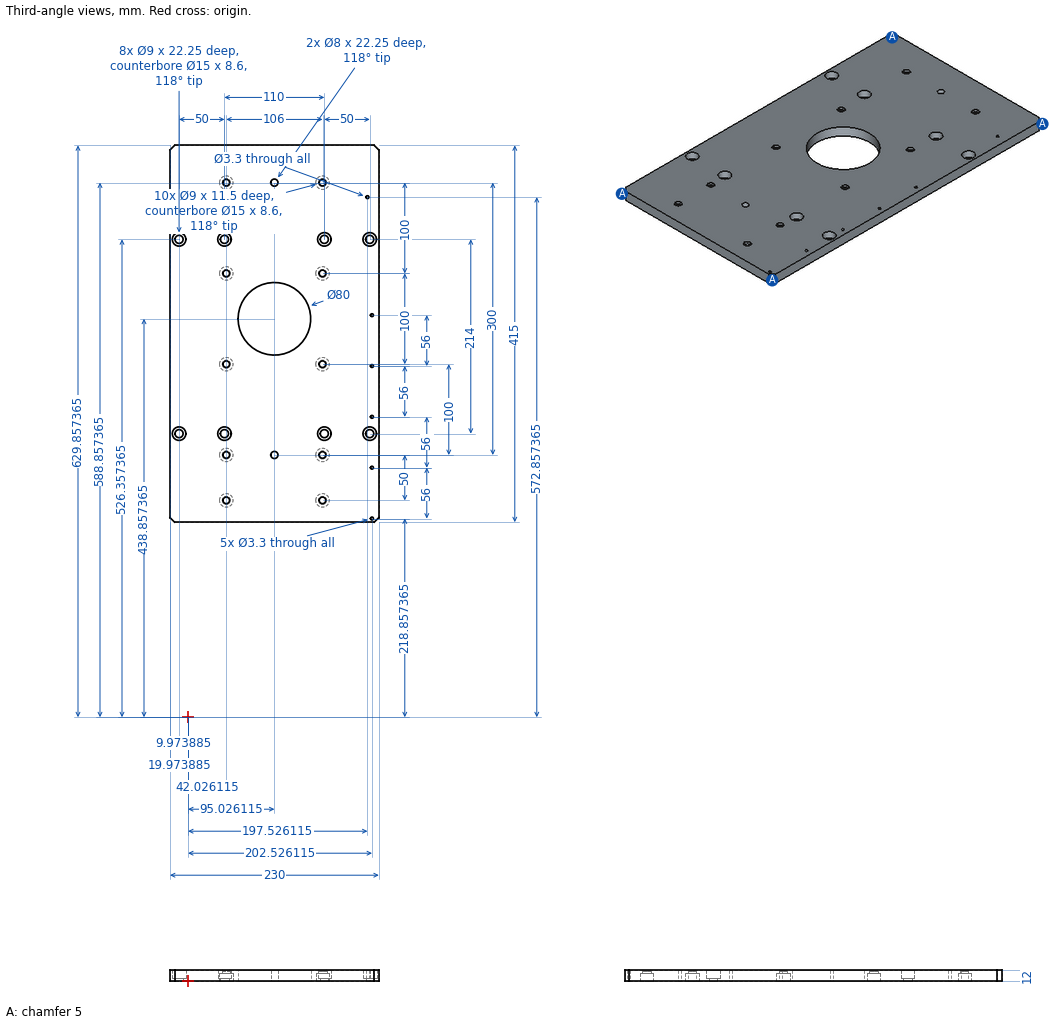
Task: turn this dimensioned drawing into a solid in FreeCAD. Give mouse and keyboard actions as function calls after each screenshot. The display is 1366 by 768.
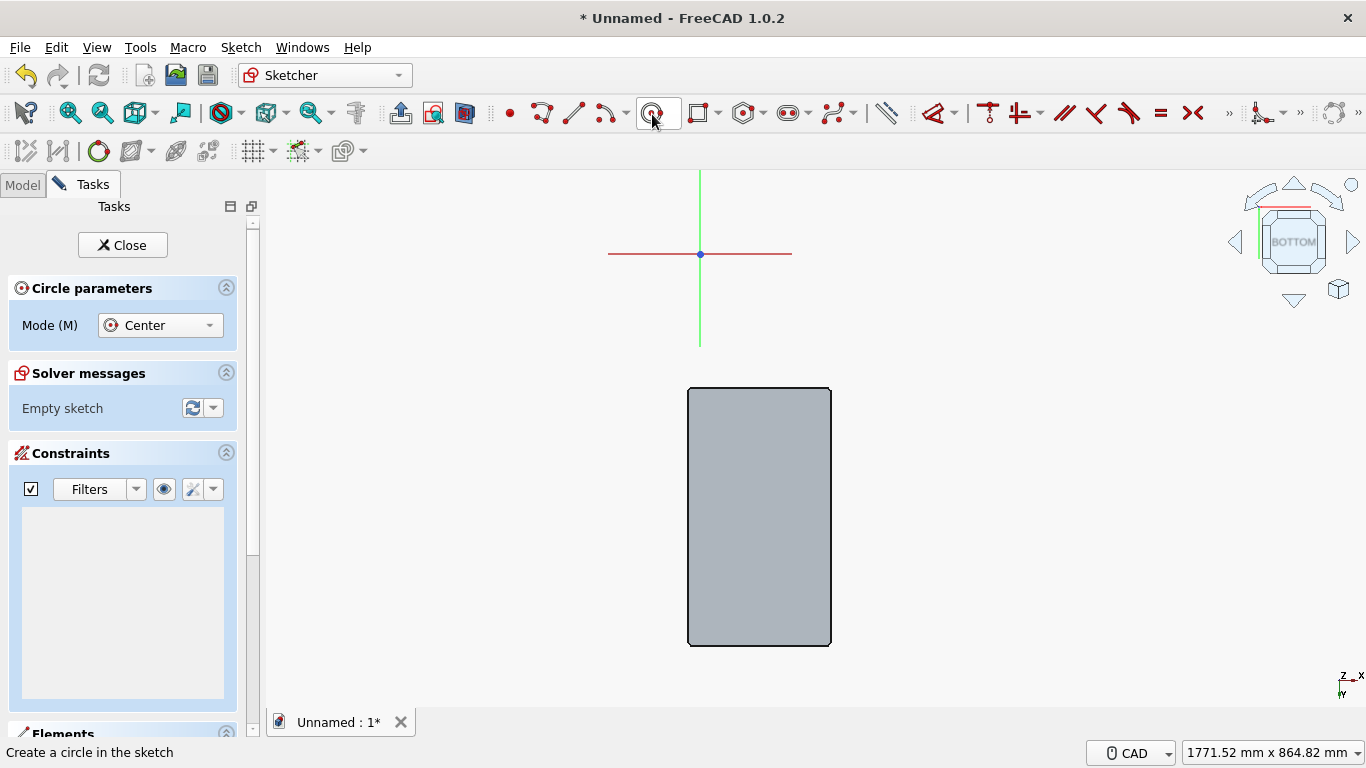
scroll(792, 620, up, 11)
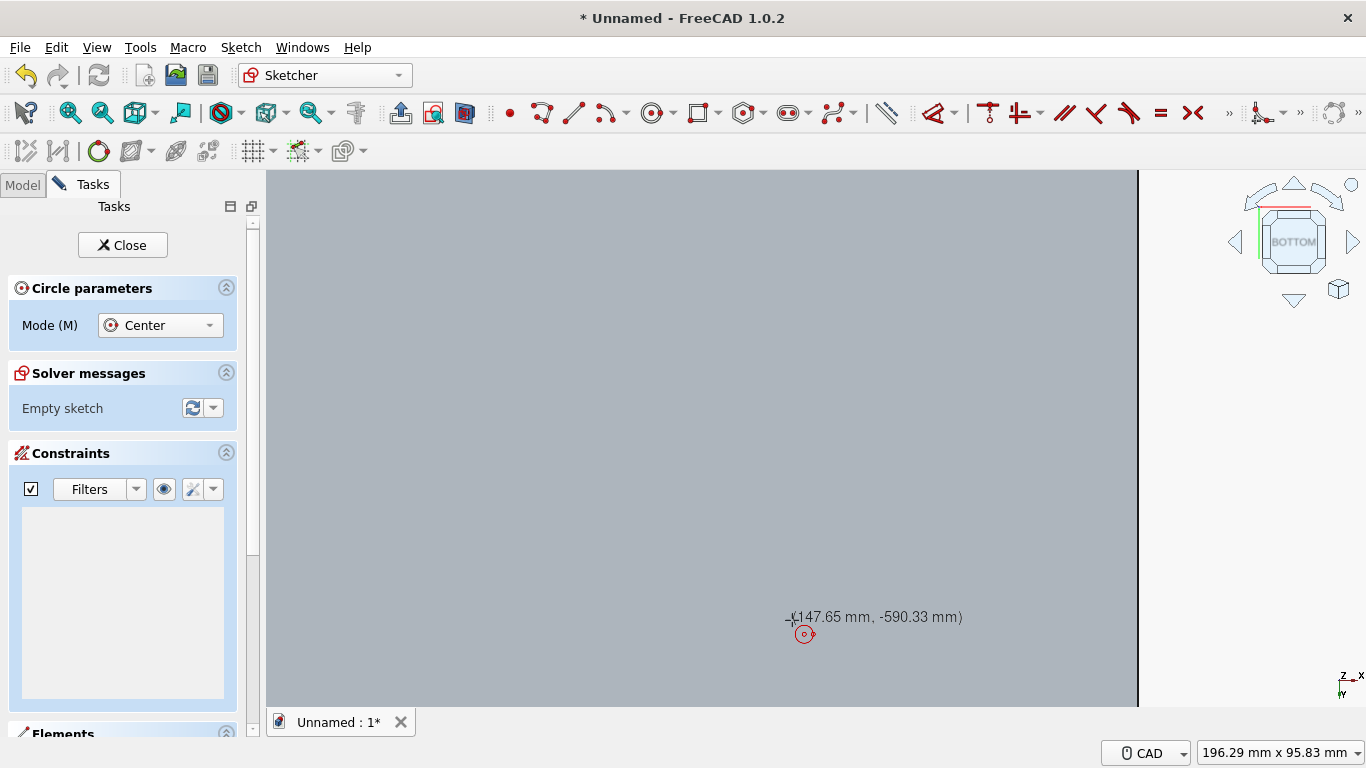
scroll(792, 621, down, 11)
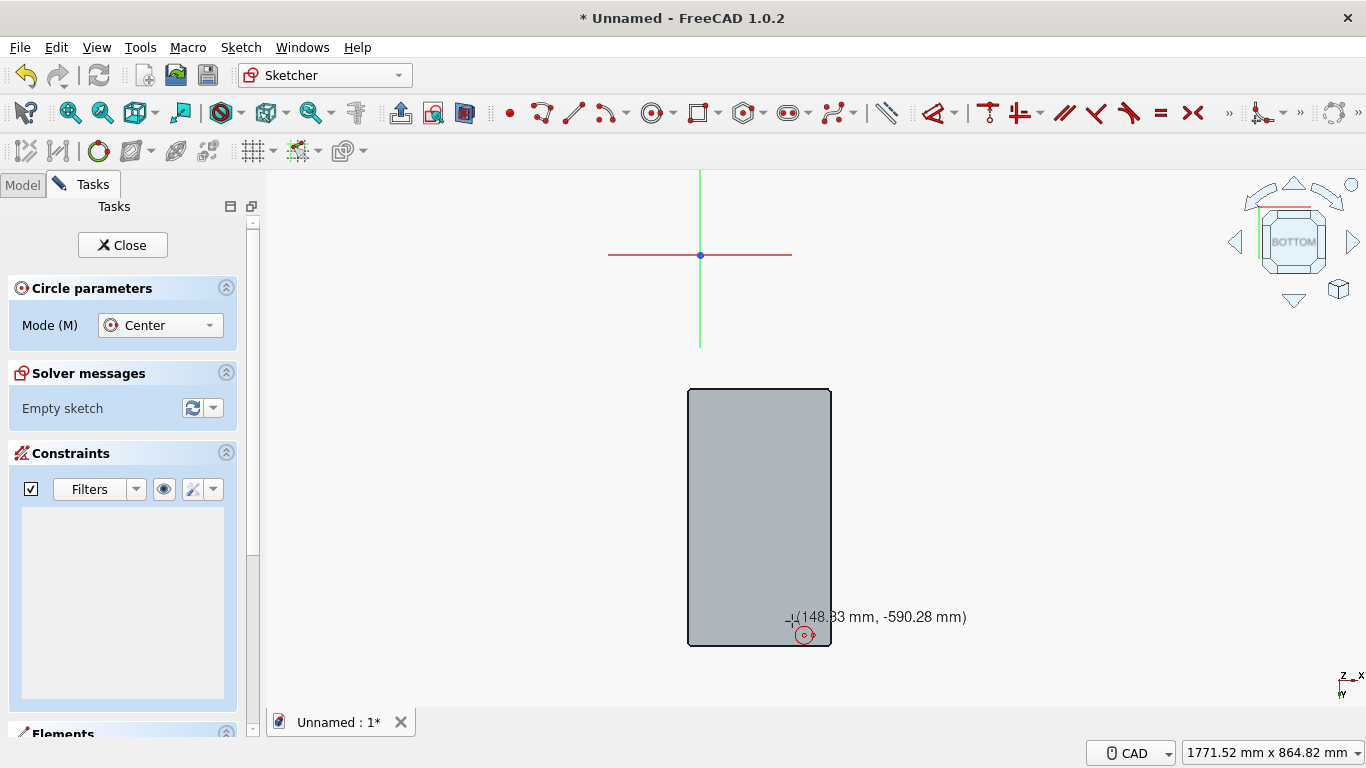
click(792, 621)
move(794, 619)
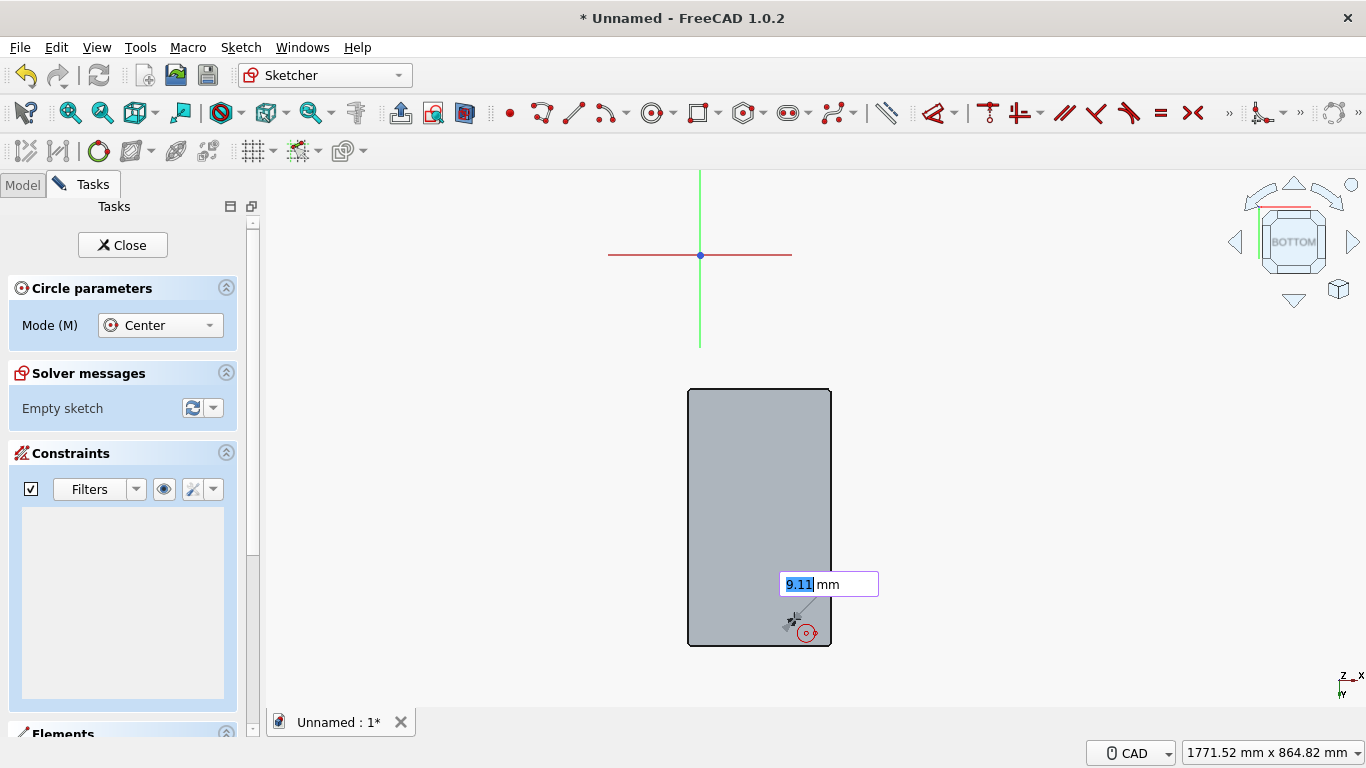
text(9)
key(Return)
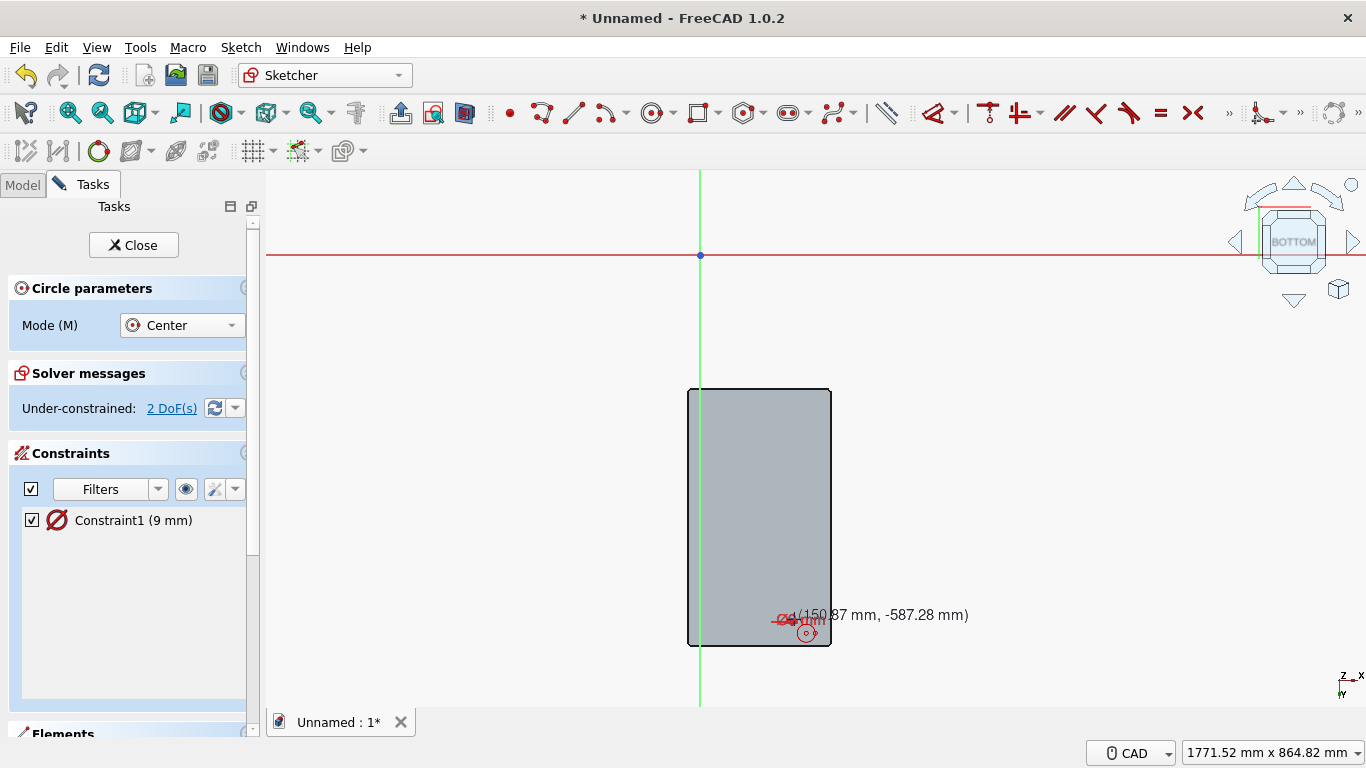
scroll(726, 621, up, 11)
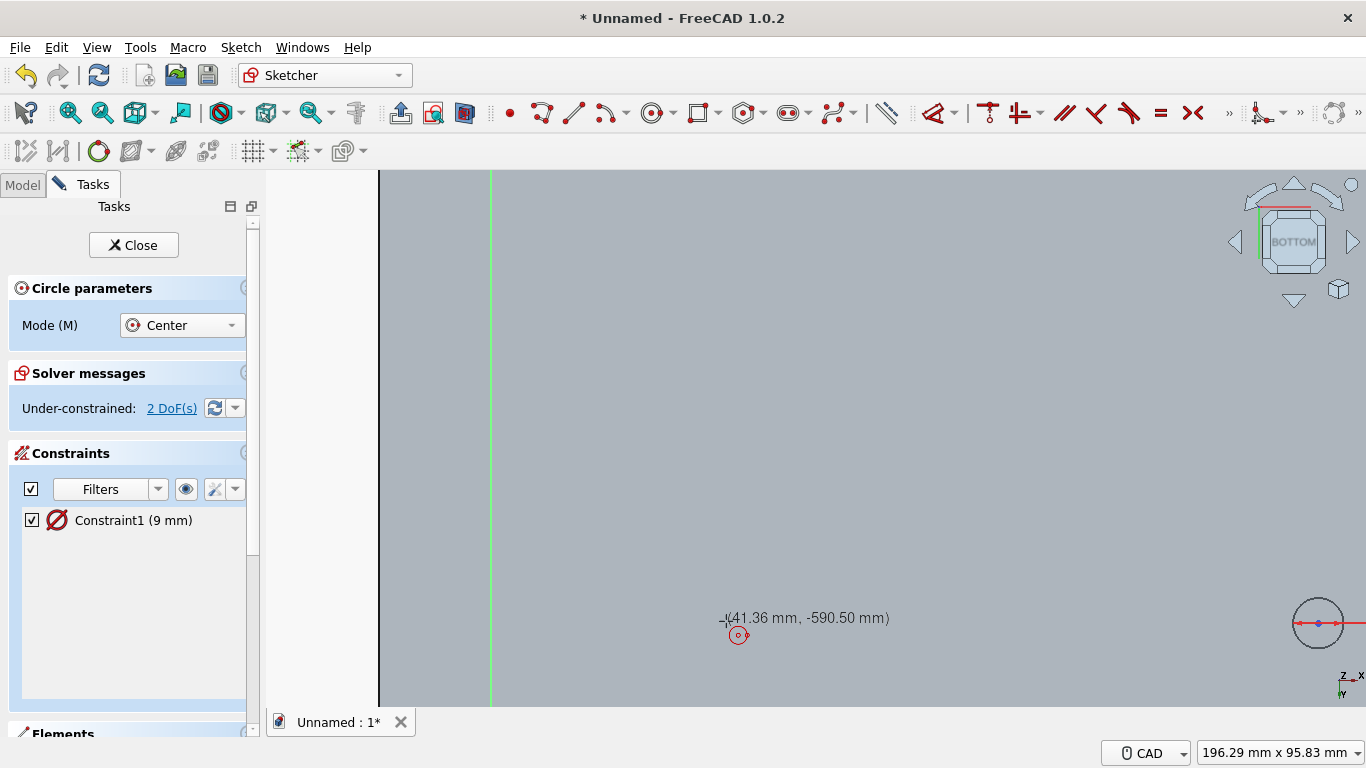
scroll(726, 621, down, 11)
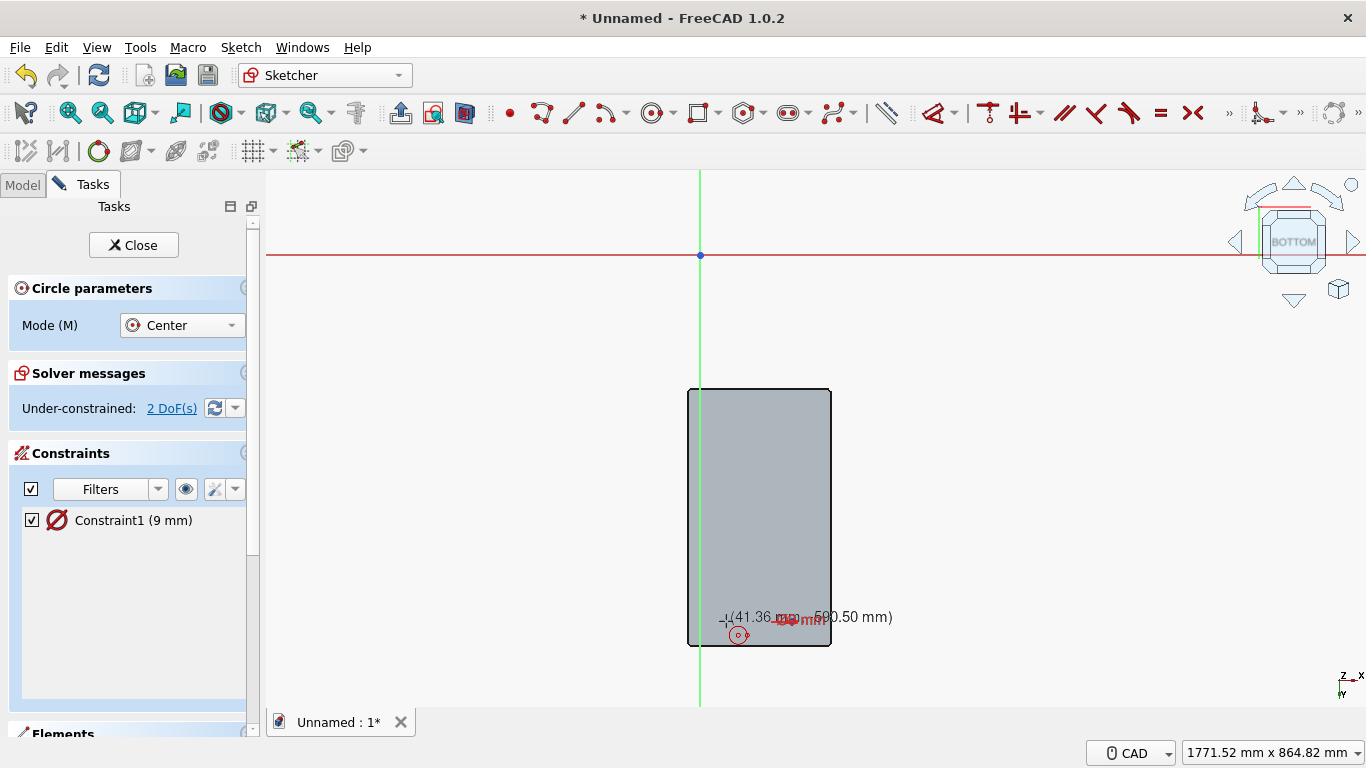
click(726, 621)
move(728, 619)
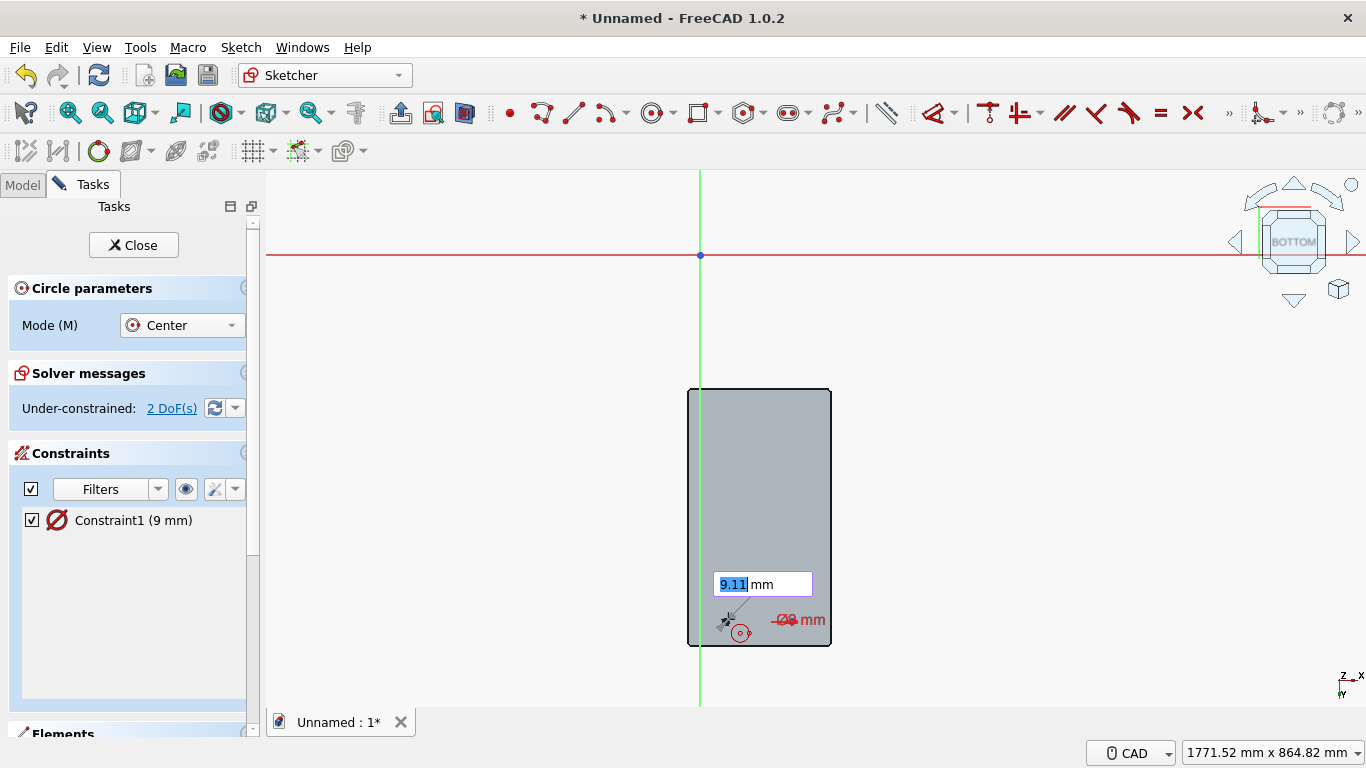
text(9)
key(Return)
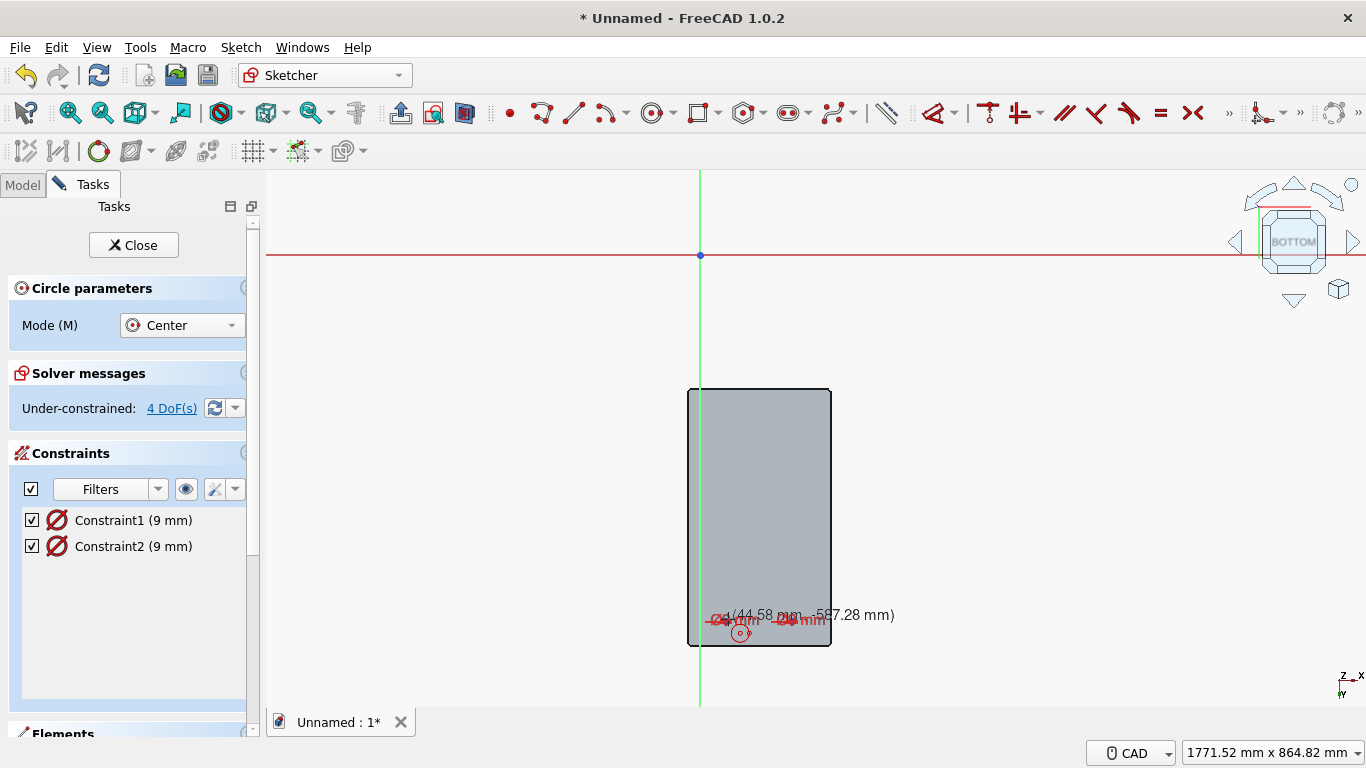
scroll(792, 559, up, 11)